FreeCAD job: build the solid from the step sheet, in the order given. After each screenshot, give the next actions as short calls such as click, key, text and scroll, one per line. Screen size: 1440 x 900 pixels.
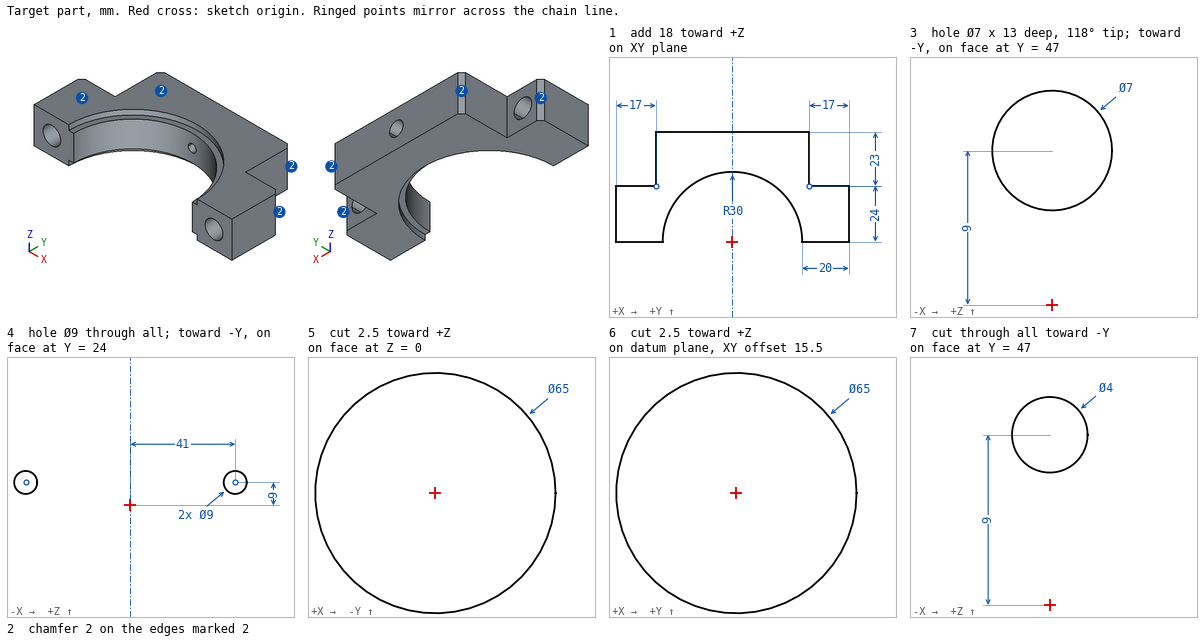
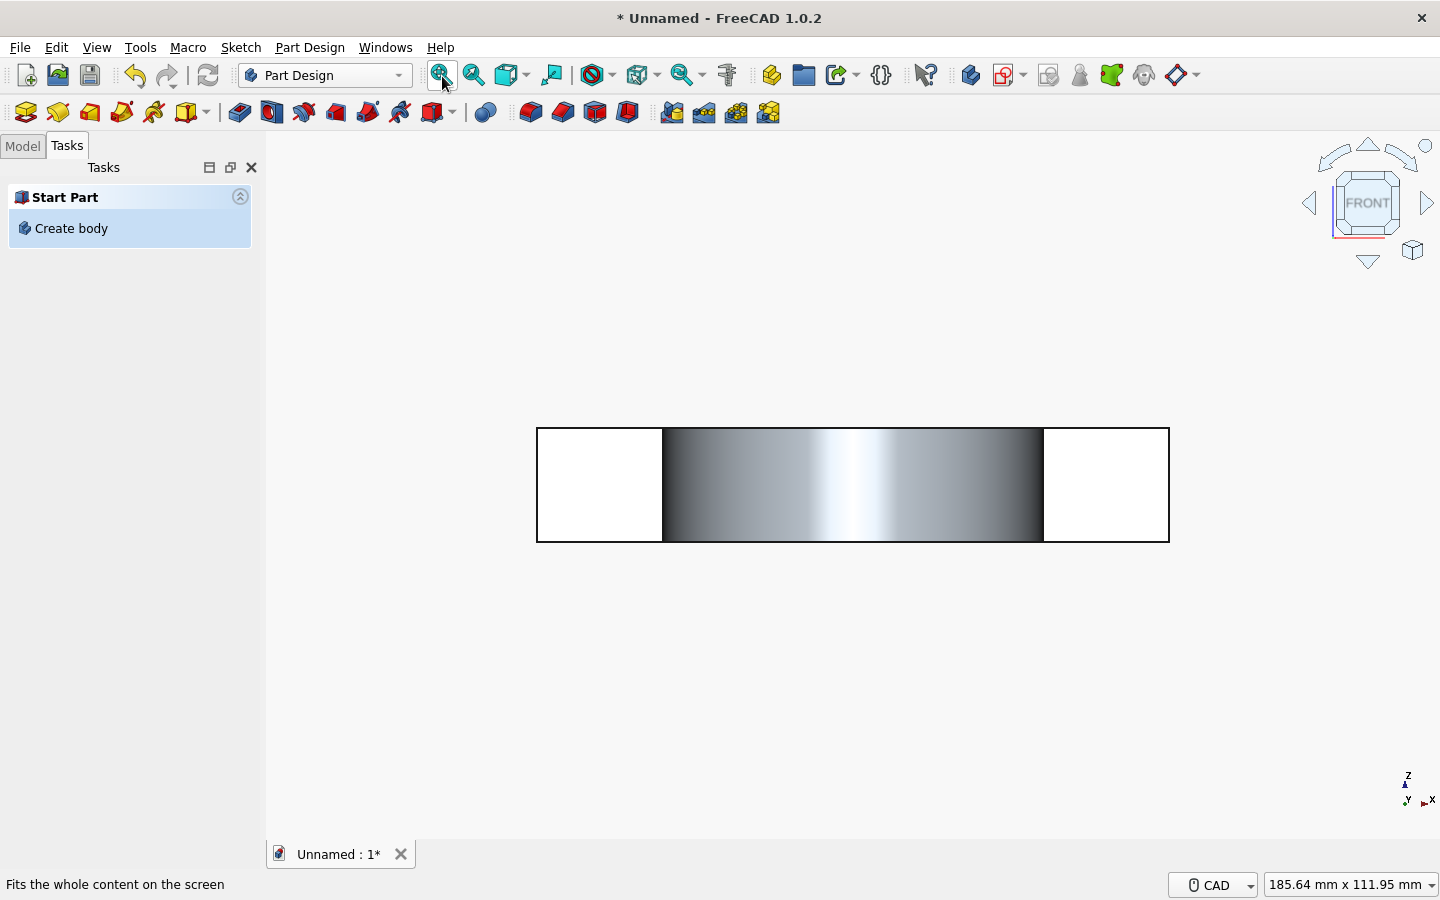
key(3)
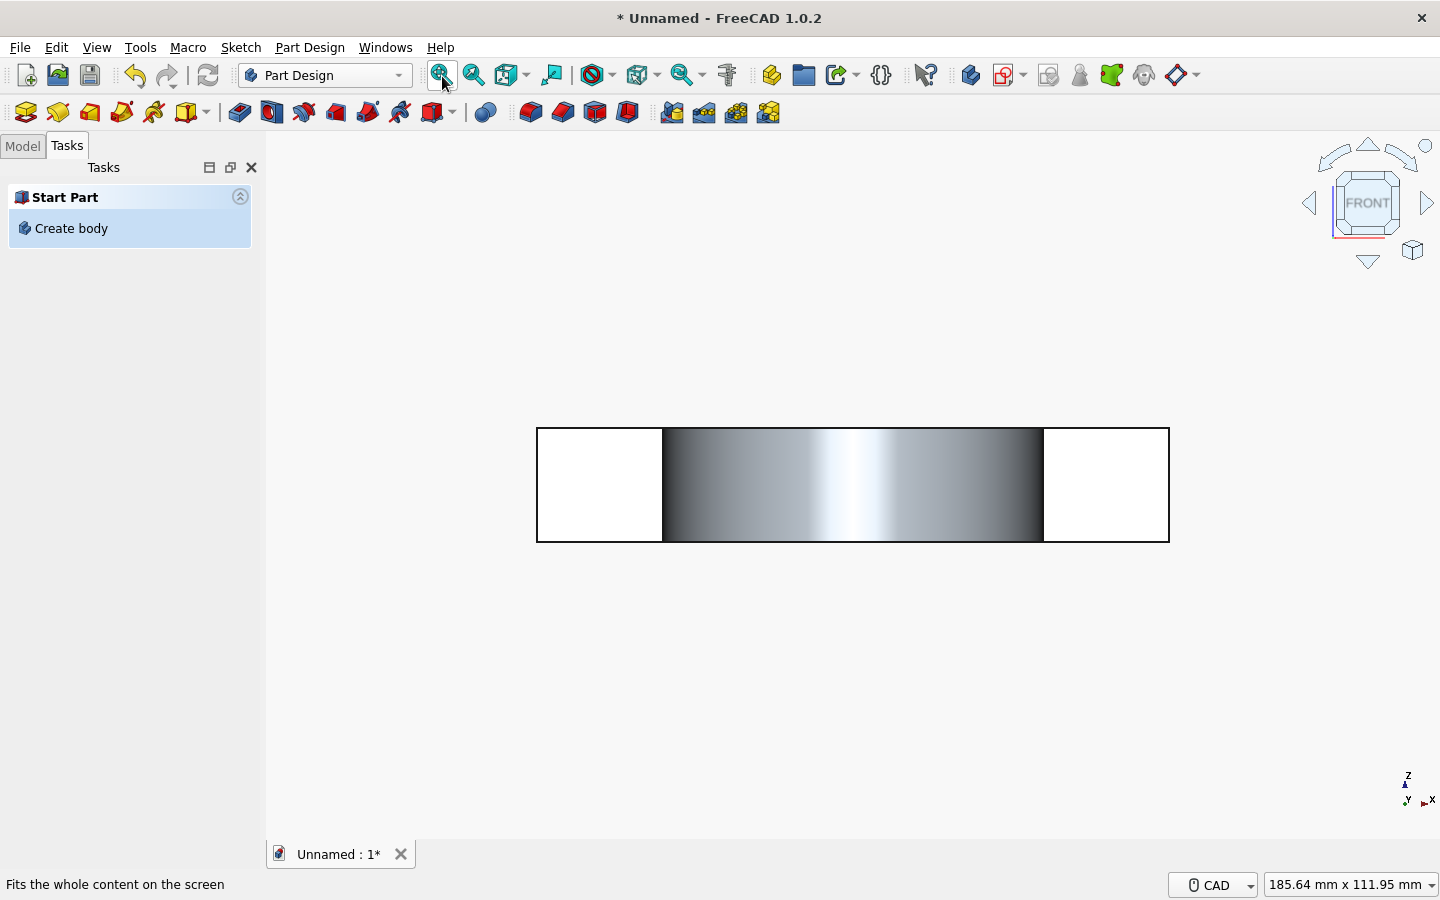
click(442, 76)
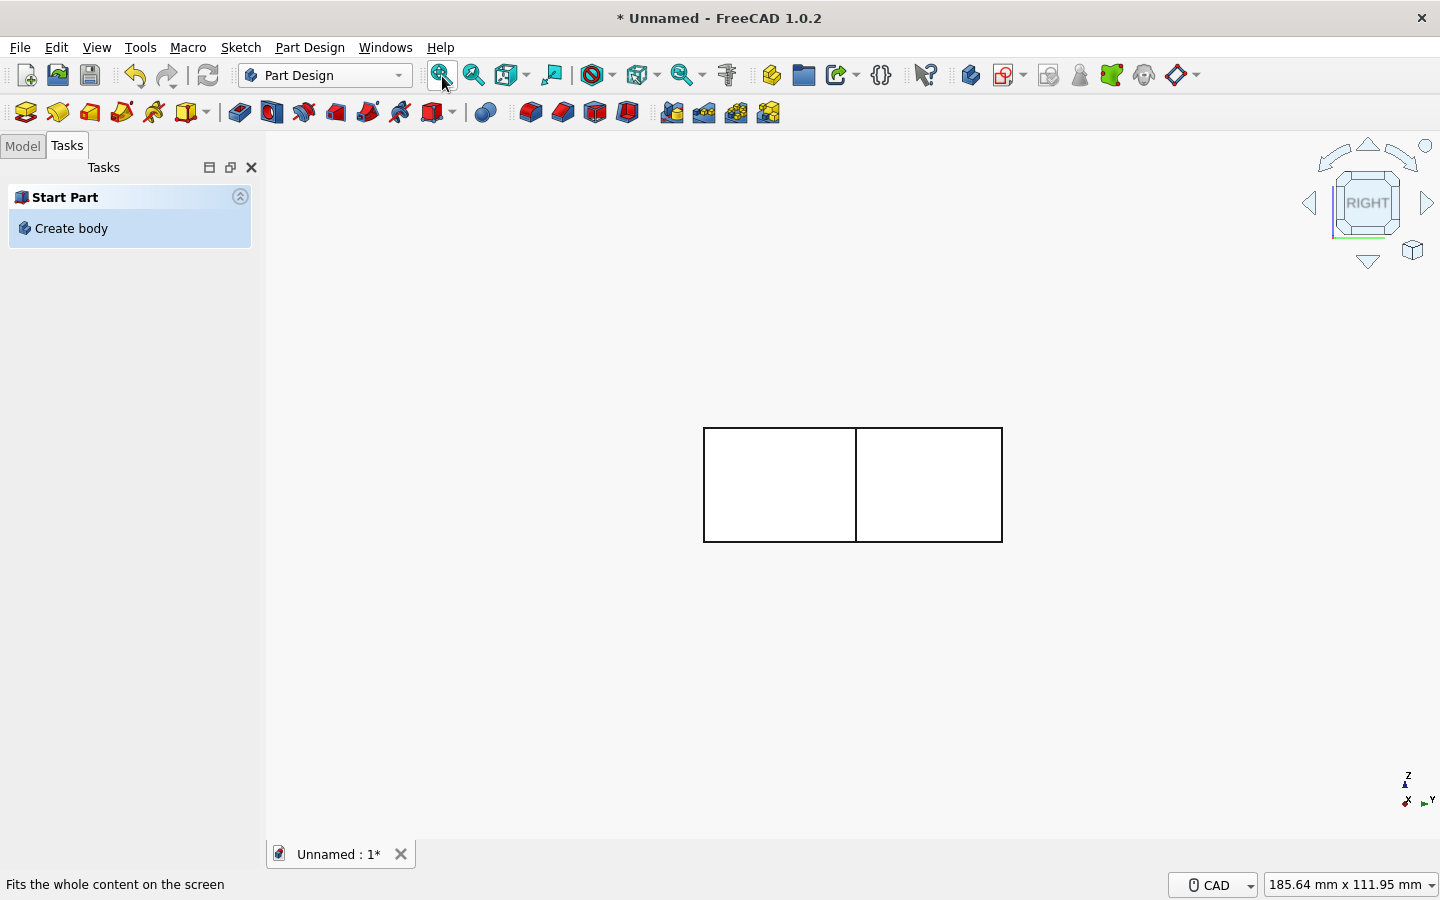
click(1002, 484)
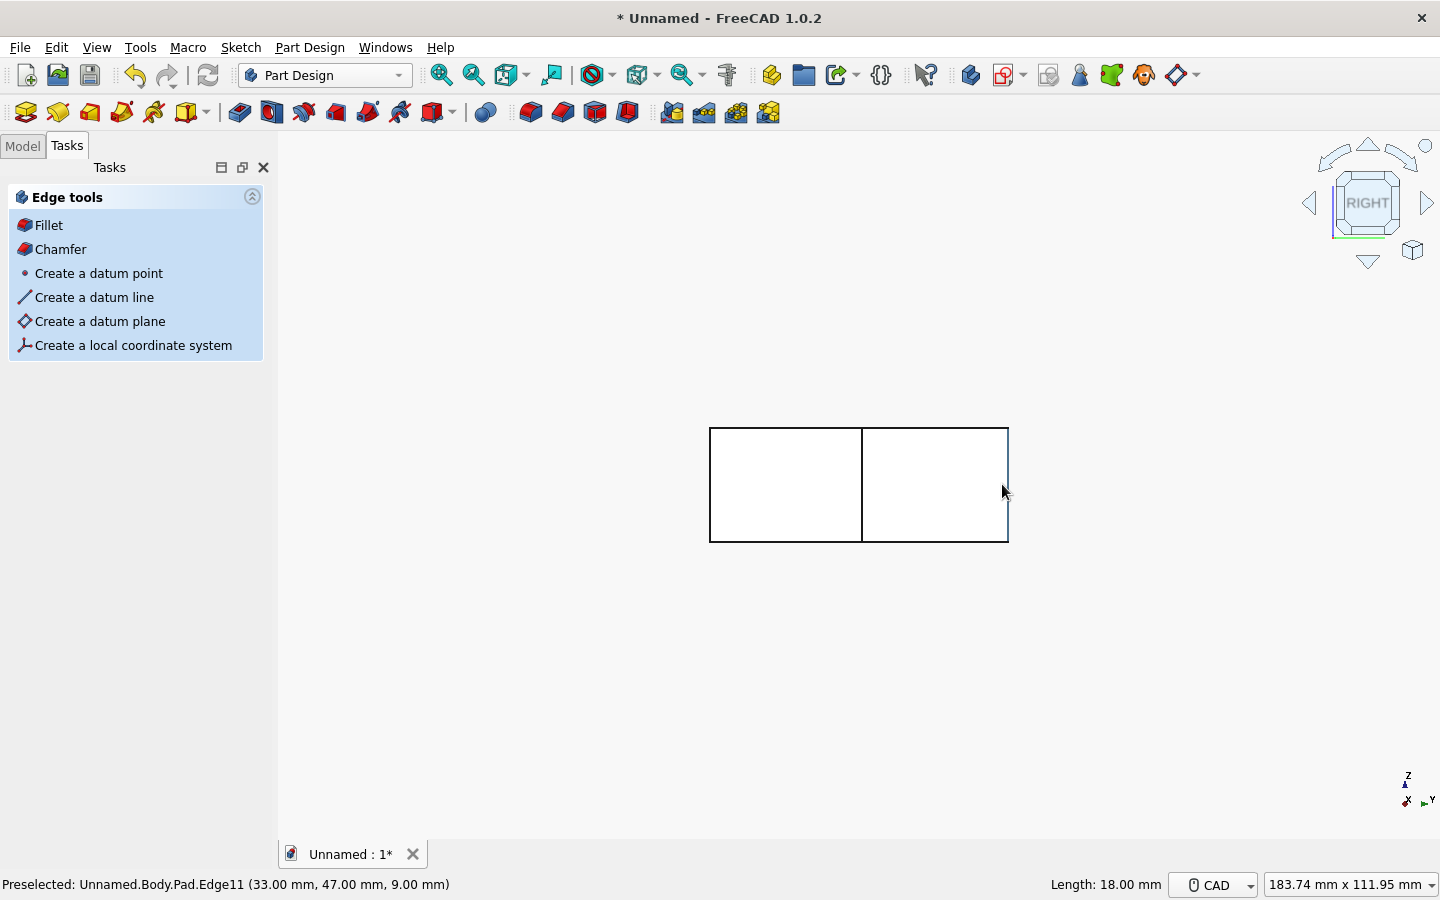
click(862, 484, ctrl)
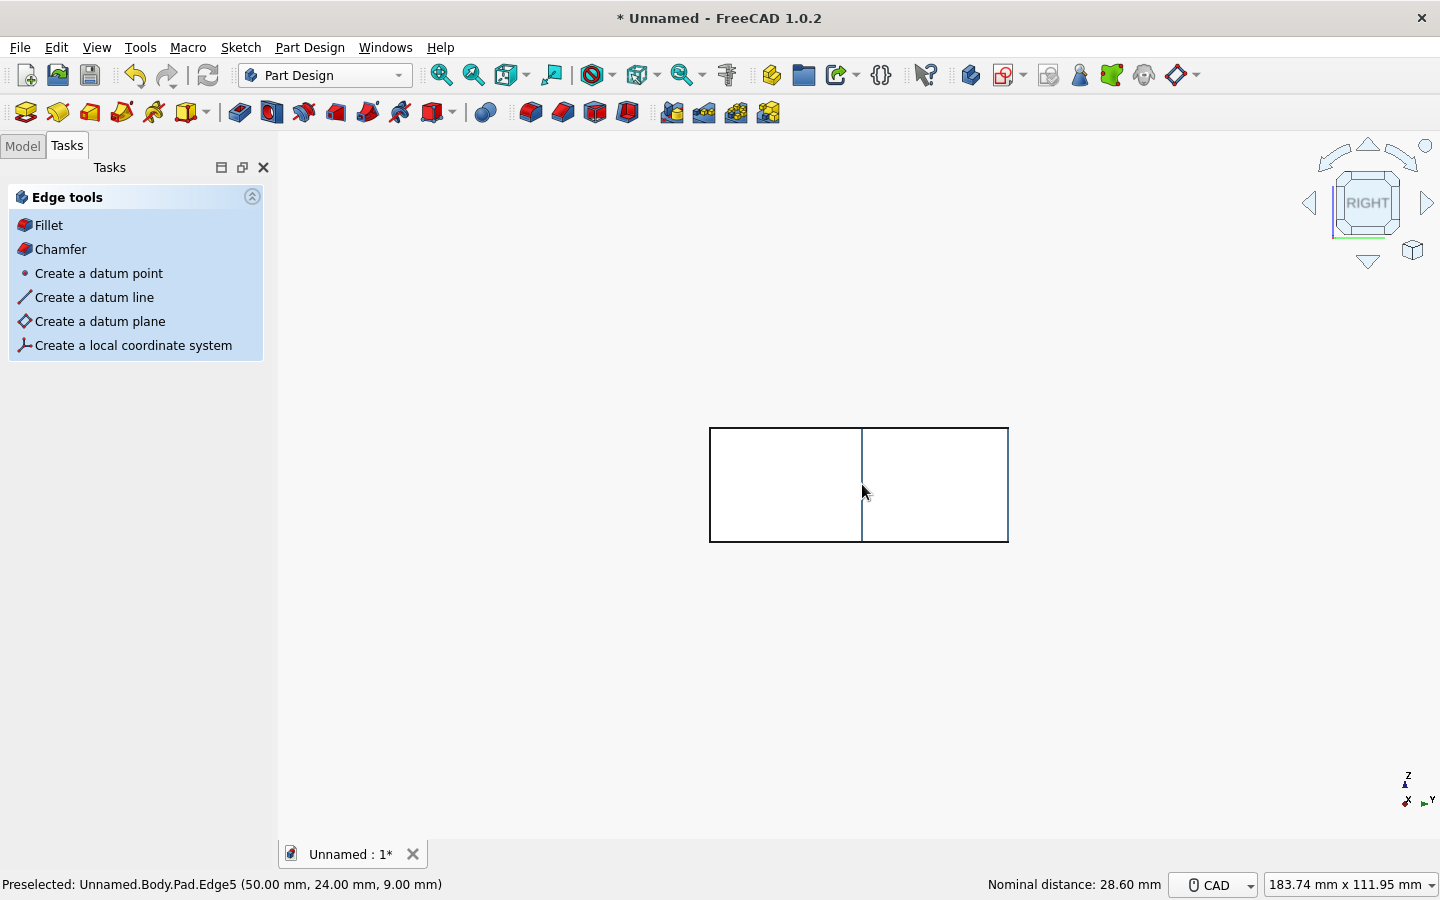
key(5)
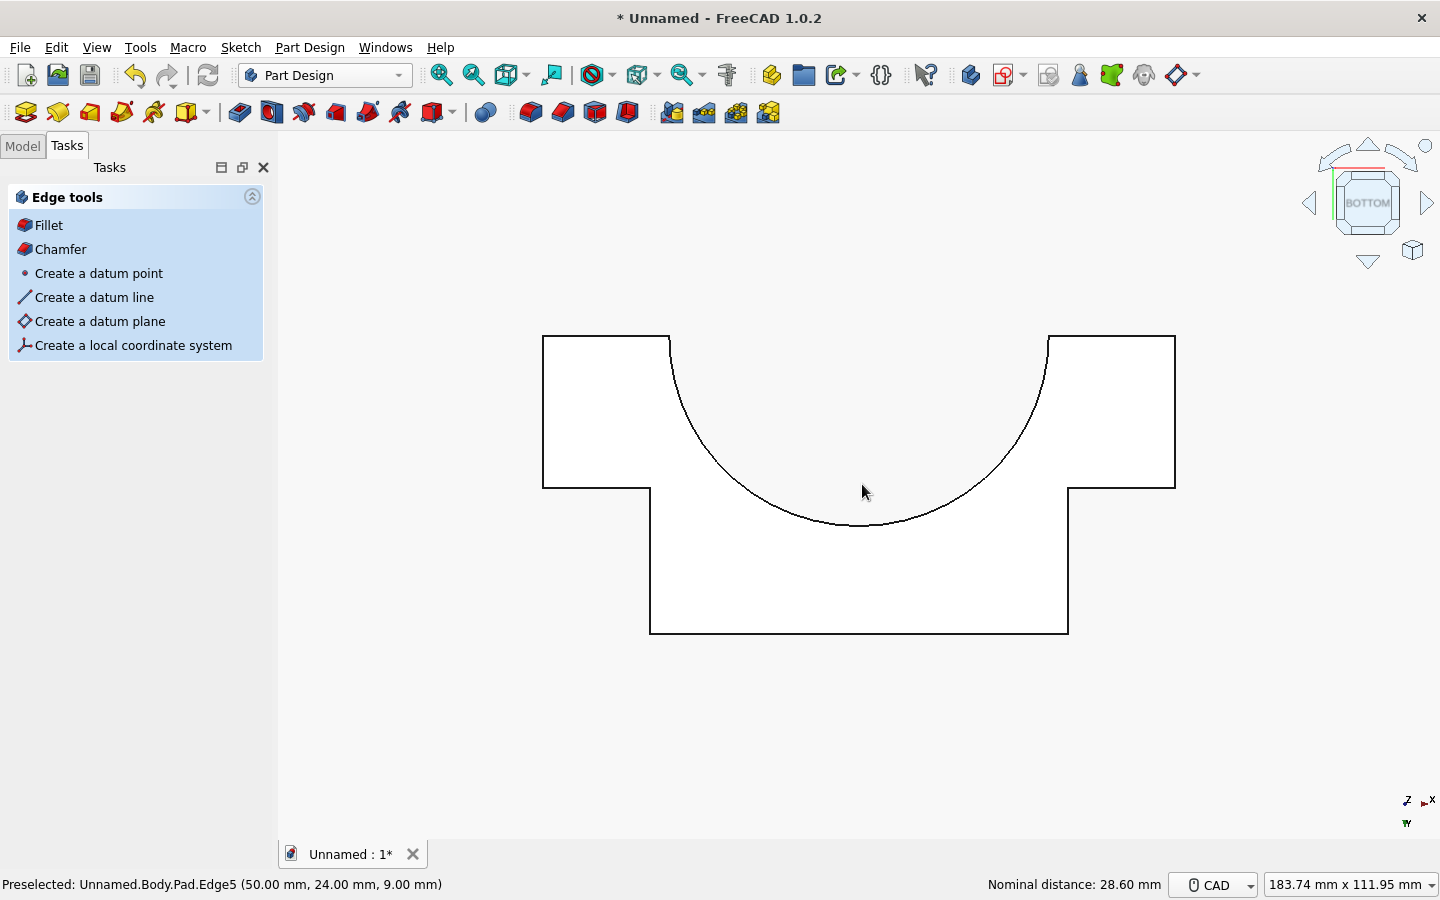
key(4)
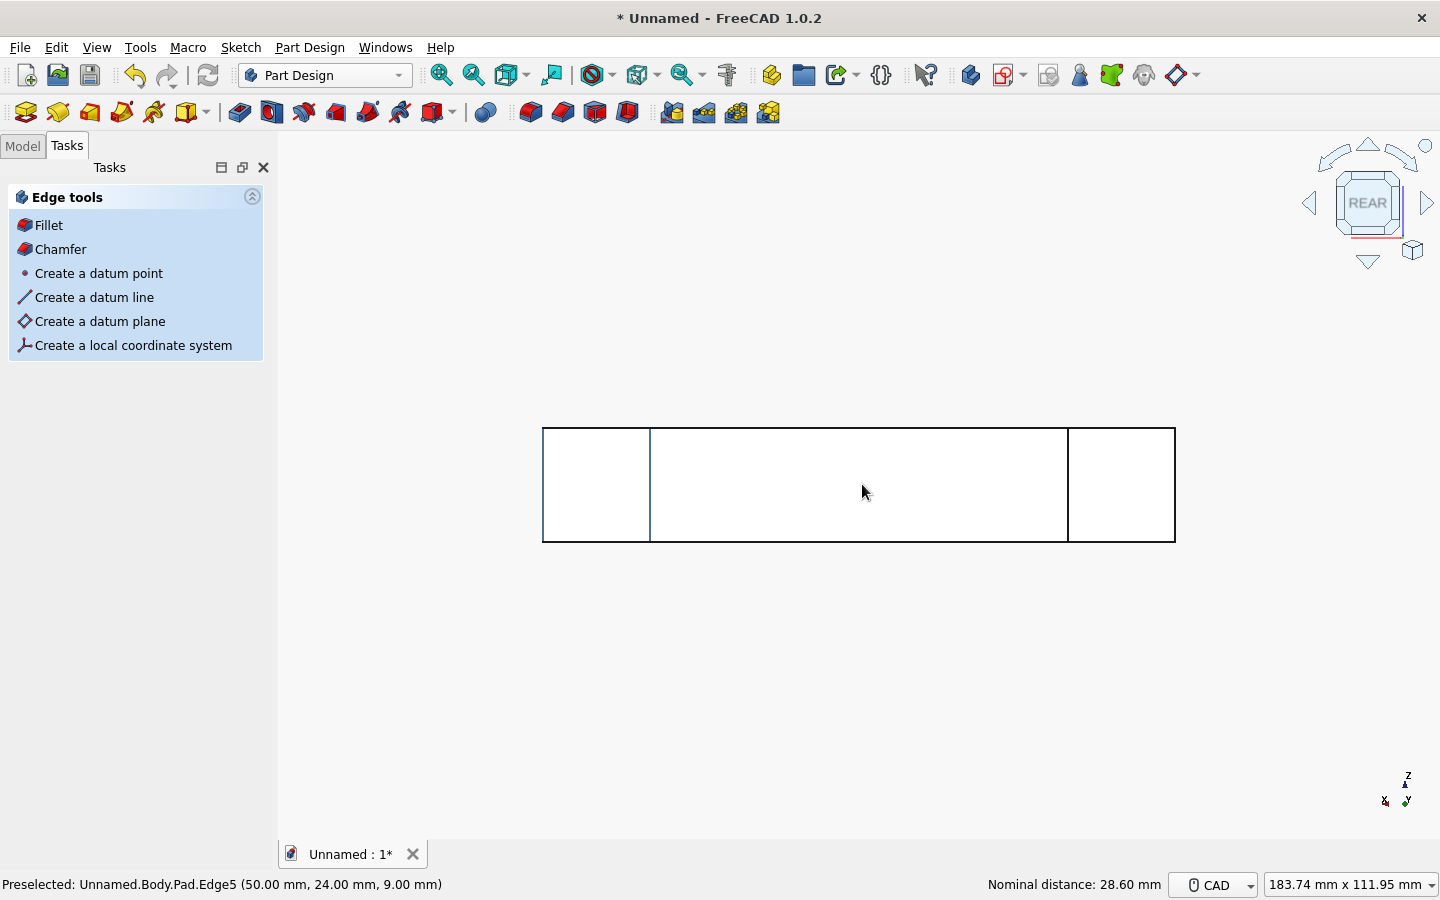
click(1175, 484, ctrl)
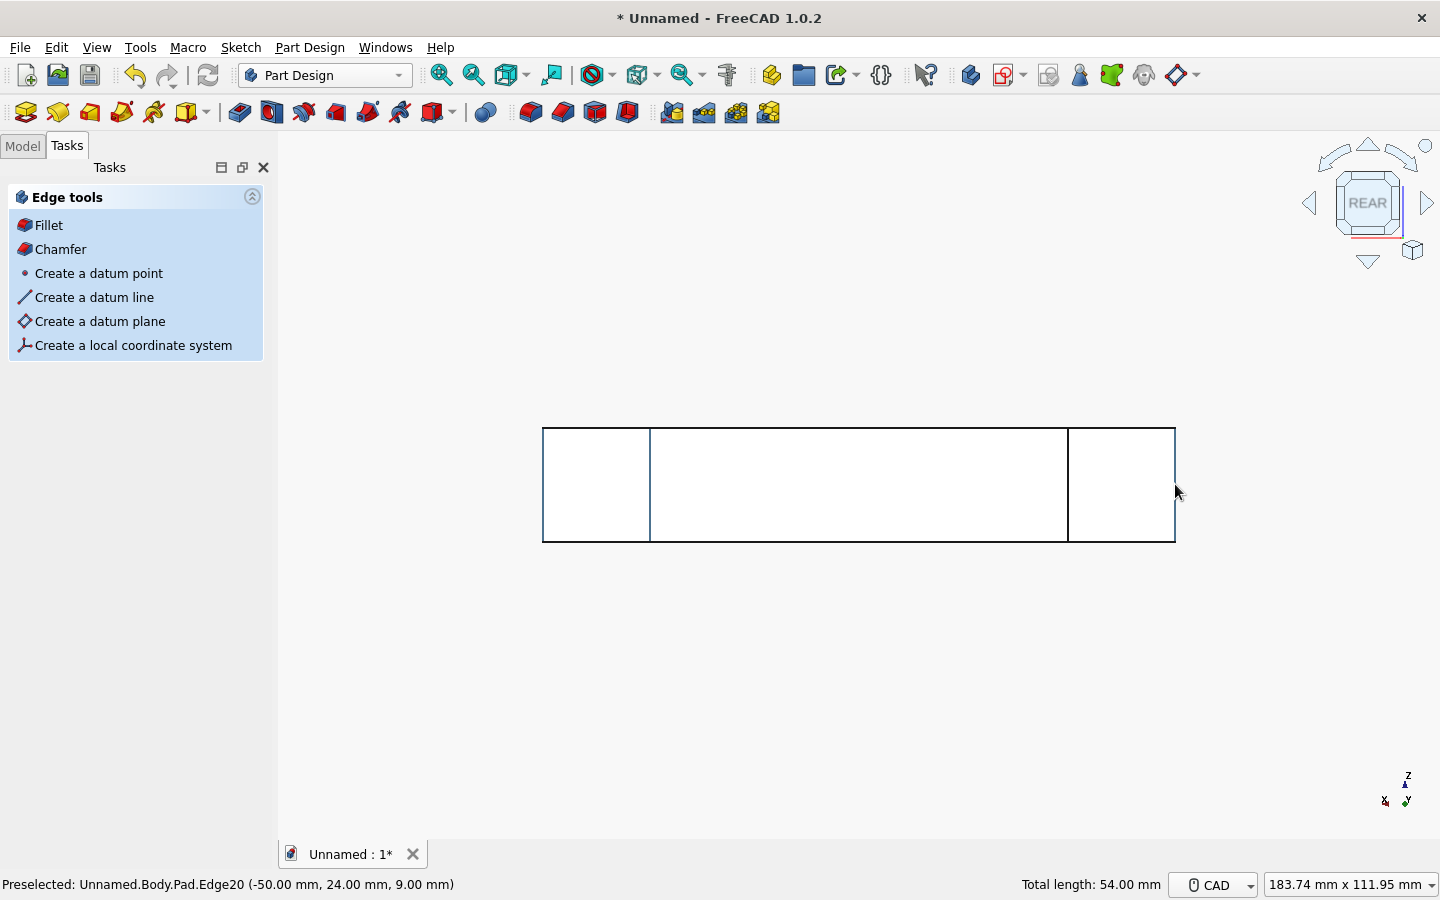
click(1068, 484, ctrl)